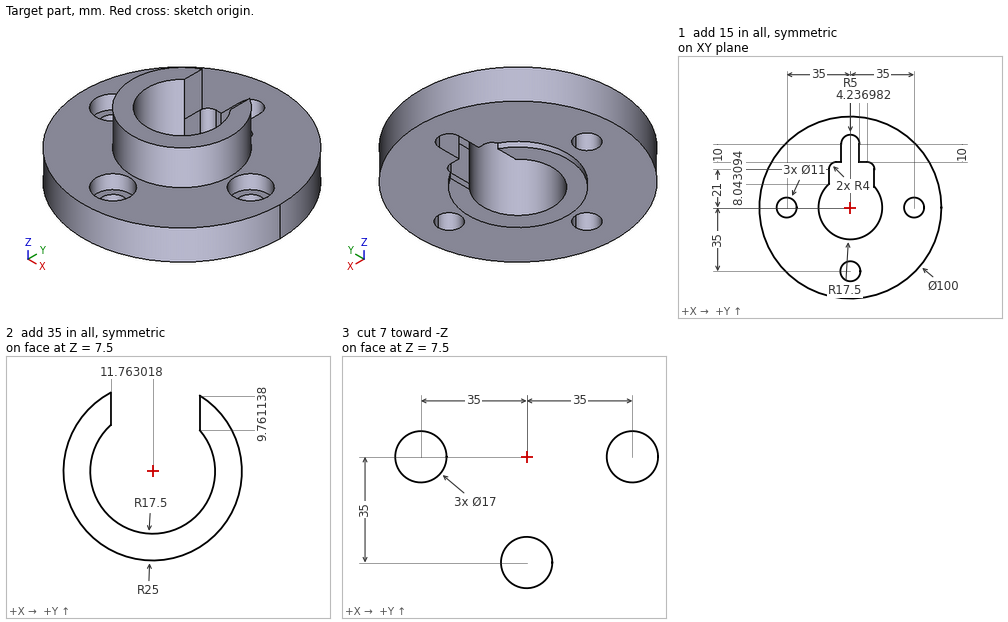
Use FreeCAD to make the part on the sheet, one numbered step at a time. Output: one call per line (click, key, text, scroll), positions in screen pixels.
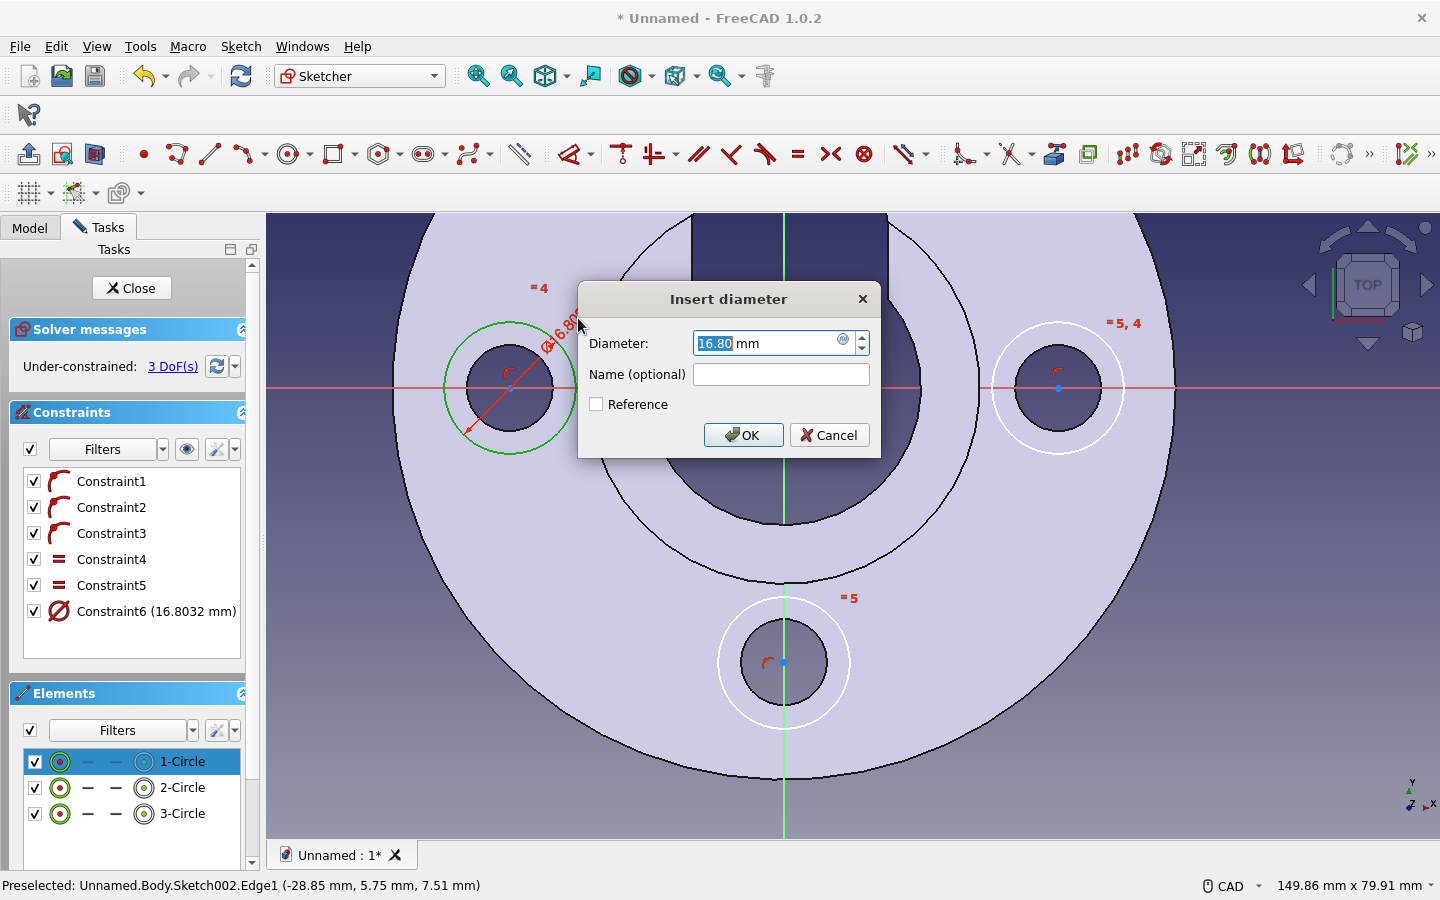
text(17)
key(Return)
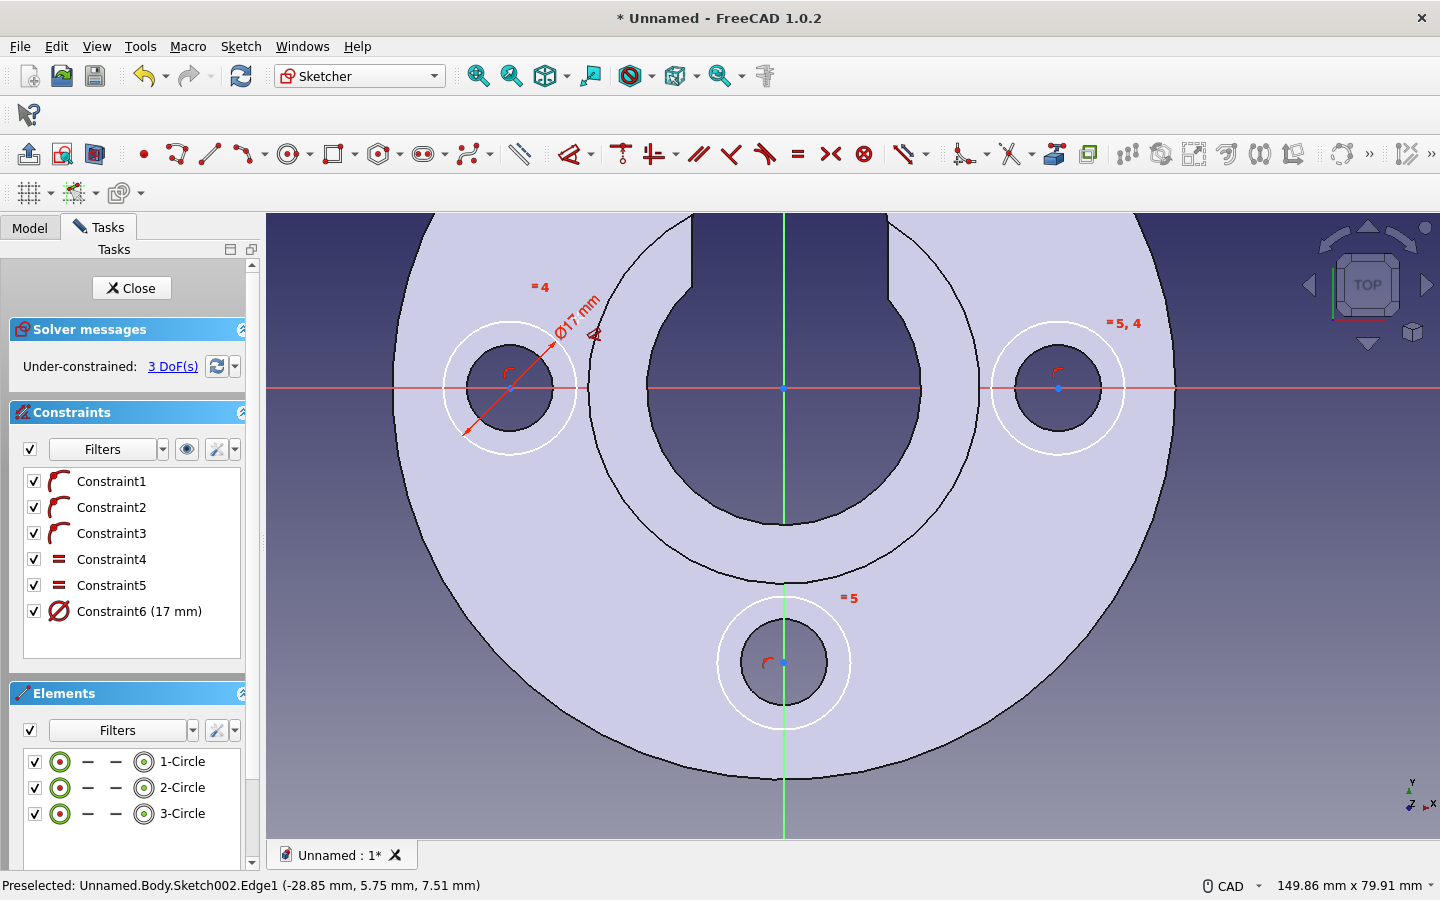
click(510, 388)
click(647, 354)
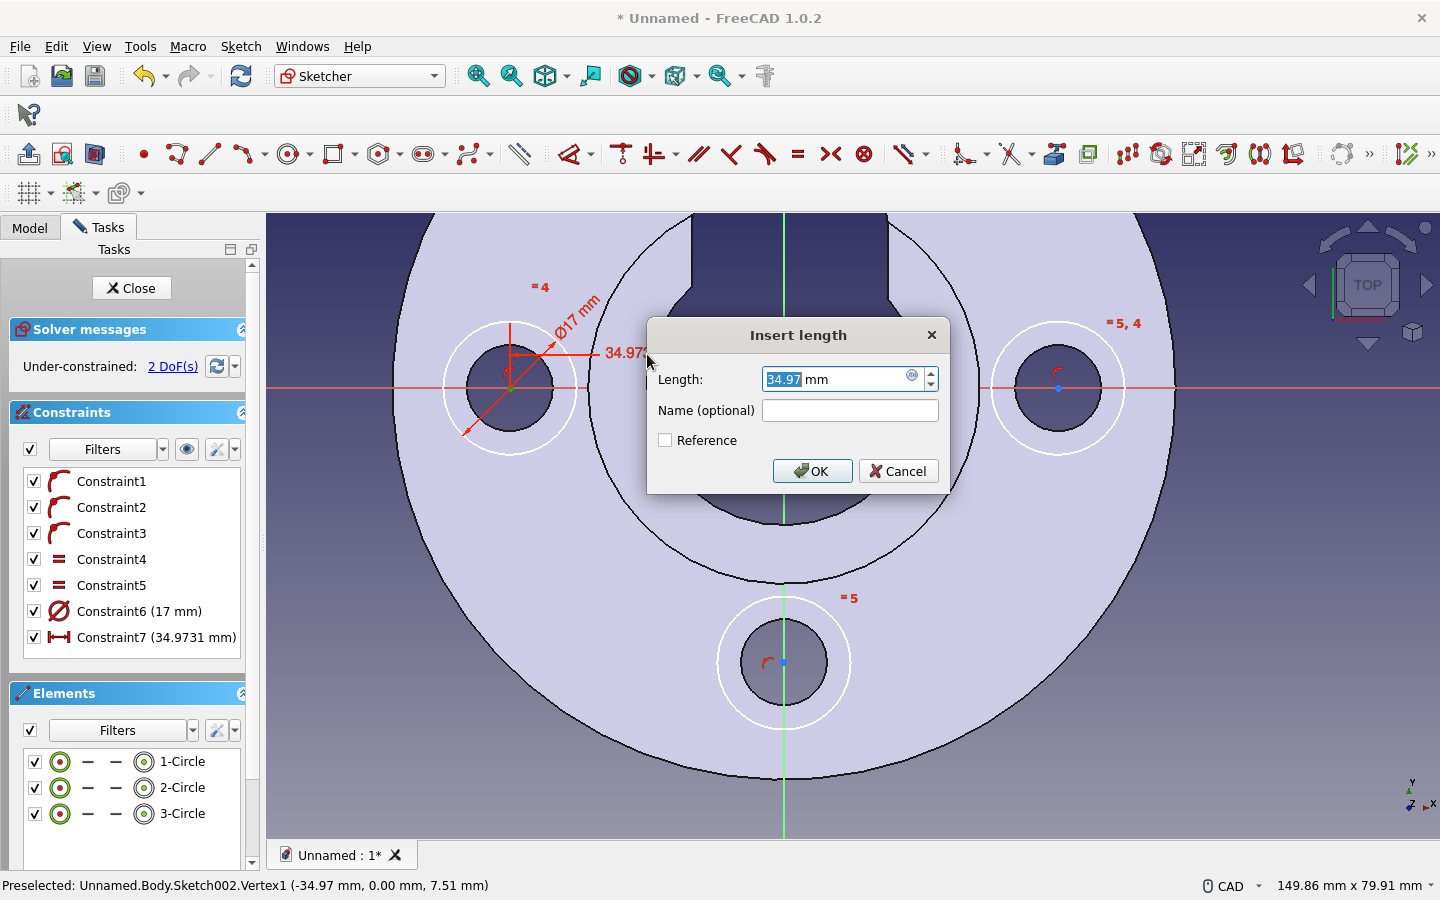
text(35)
key(Return)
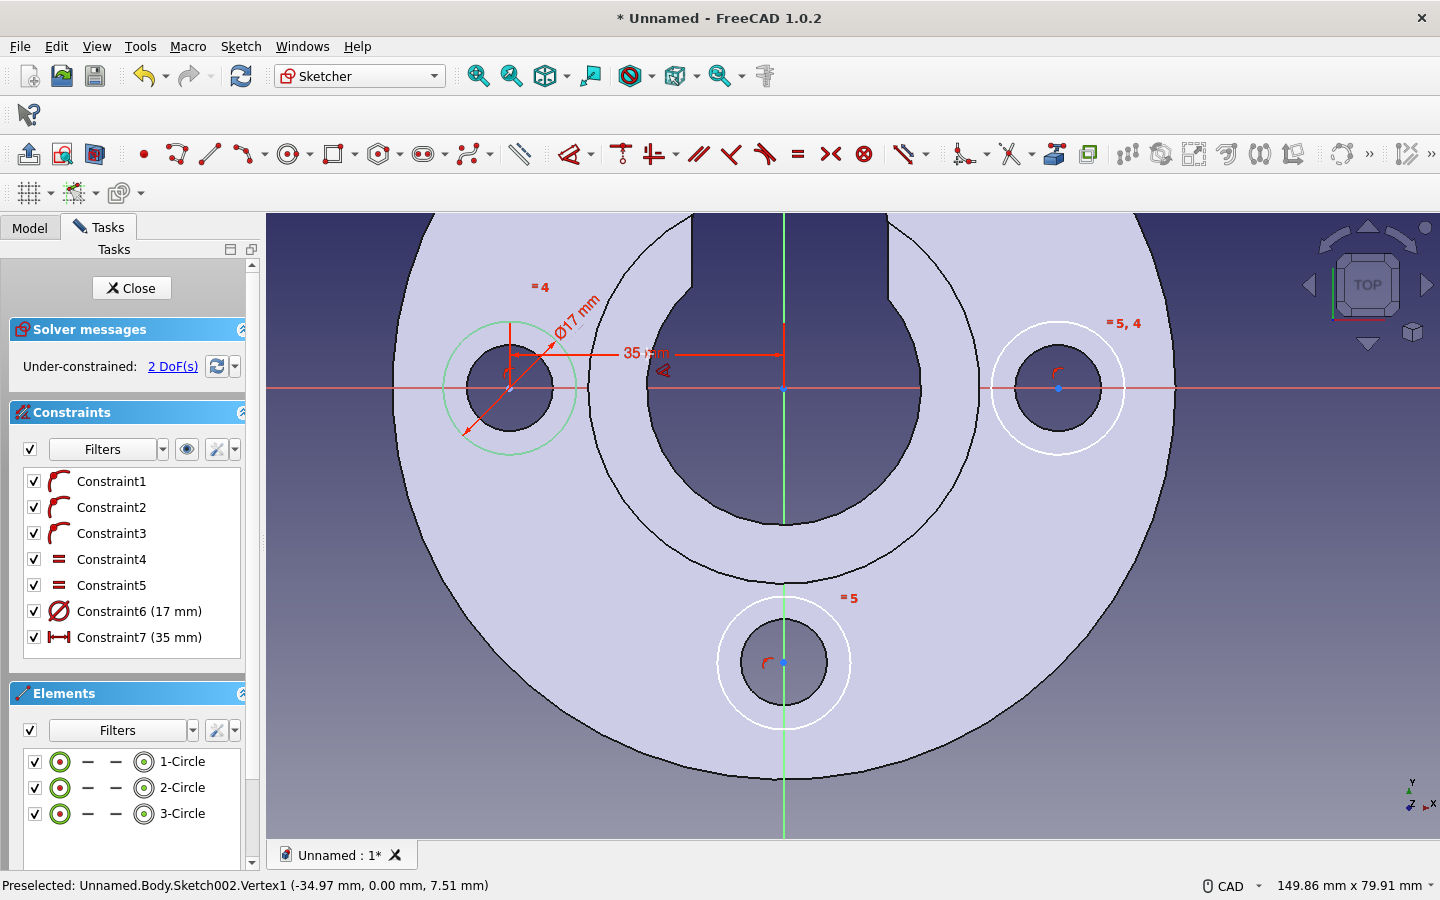
click(1058, 388)
click(921, 354)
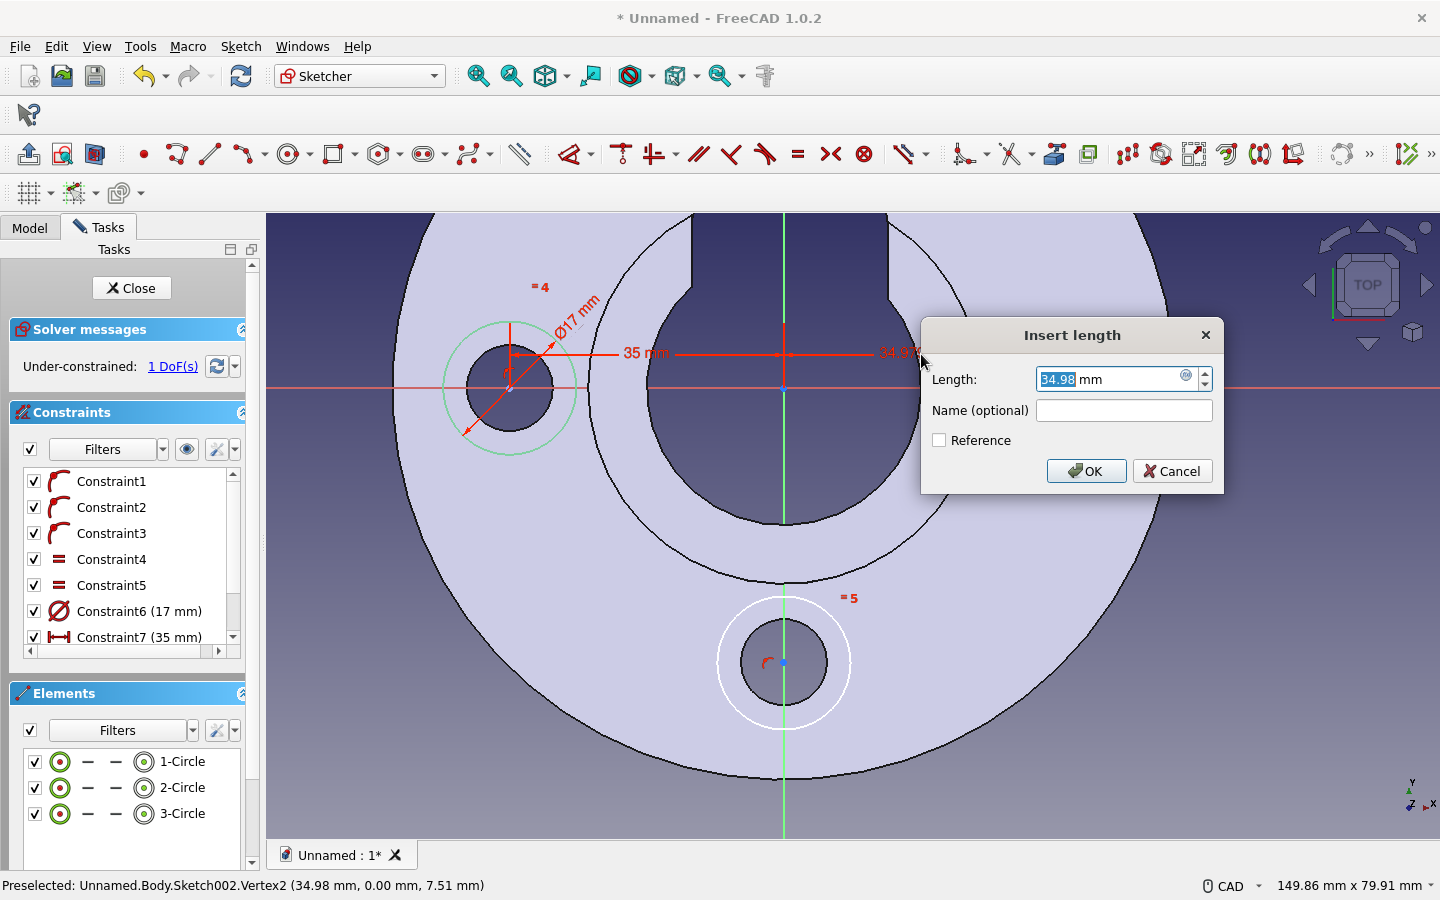
text(35)
key(Return)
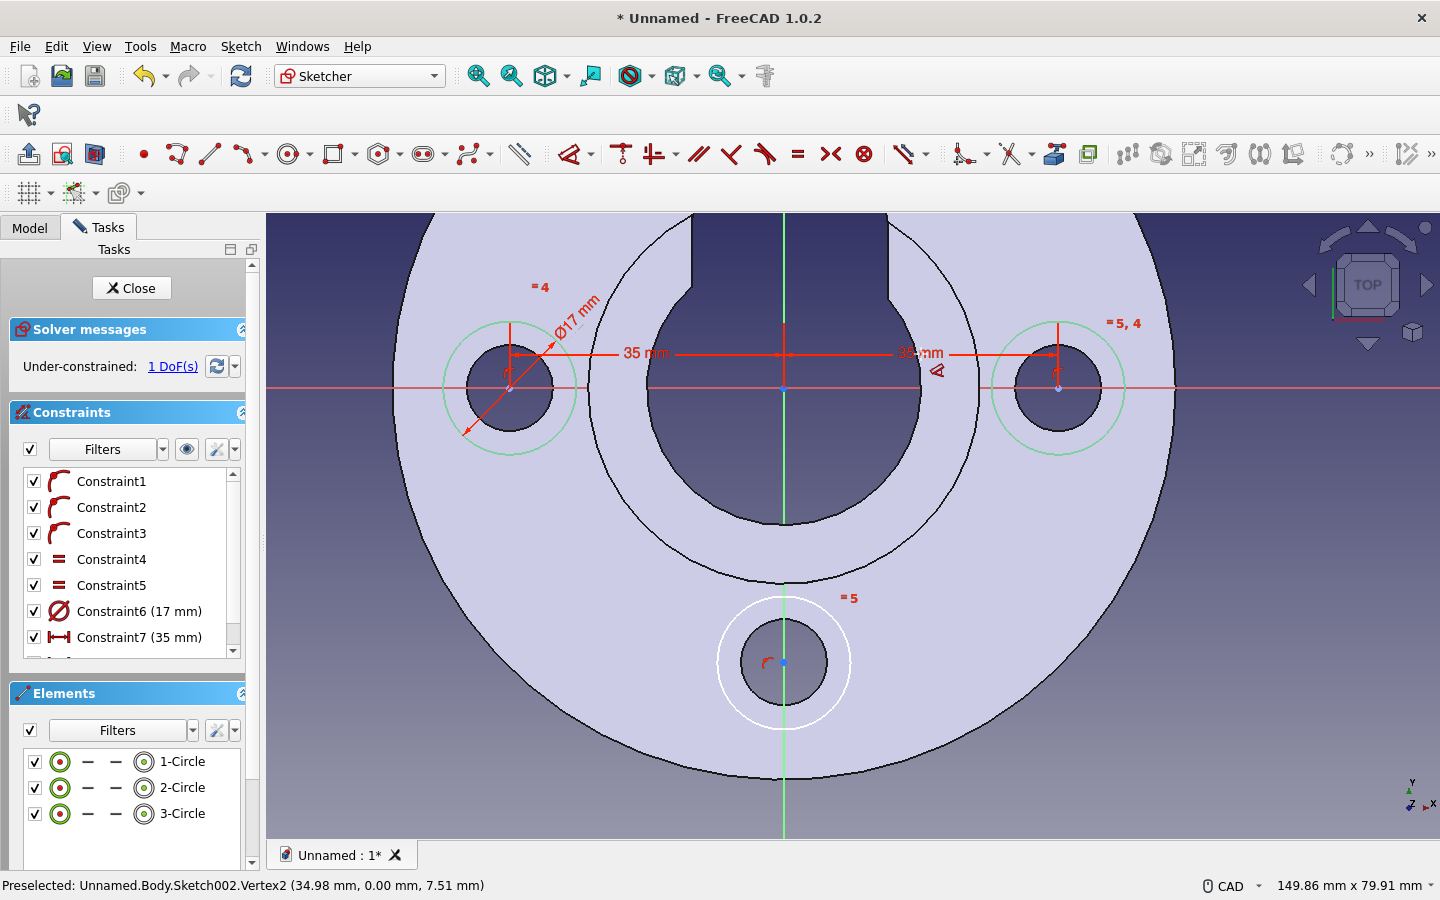
click(784, 663)
click(818, 526)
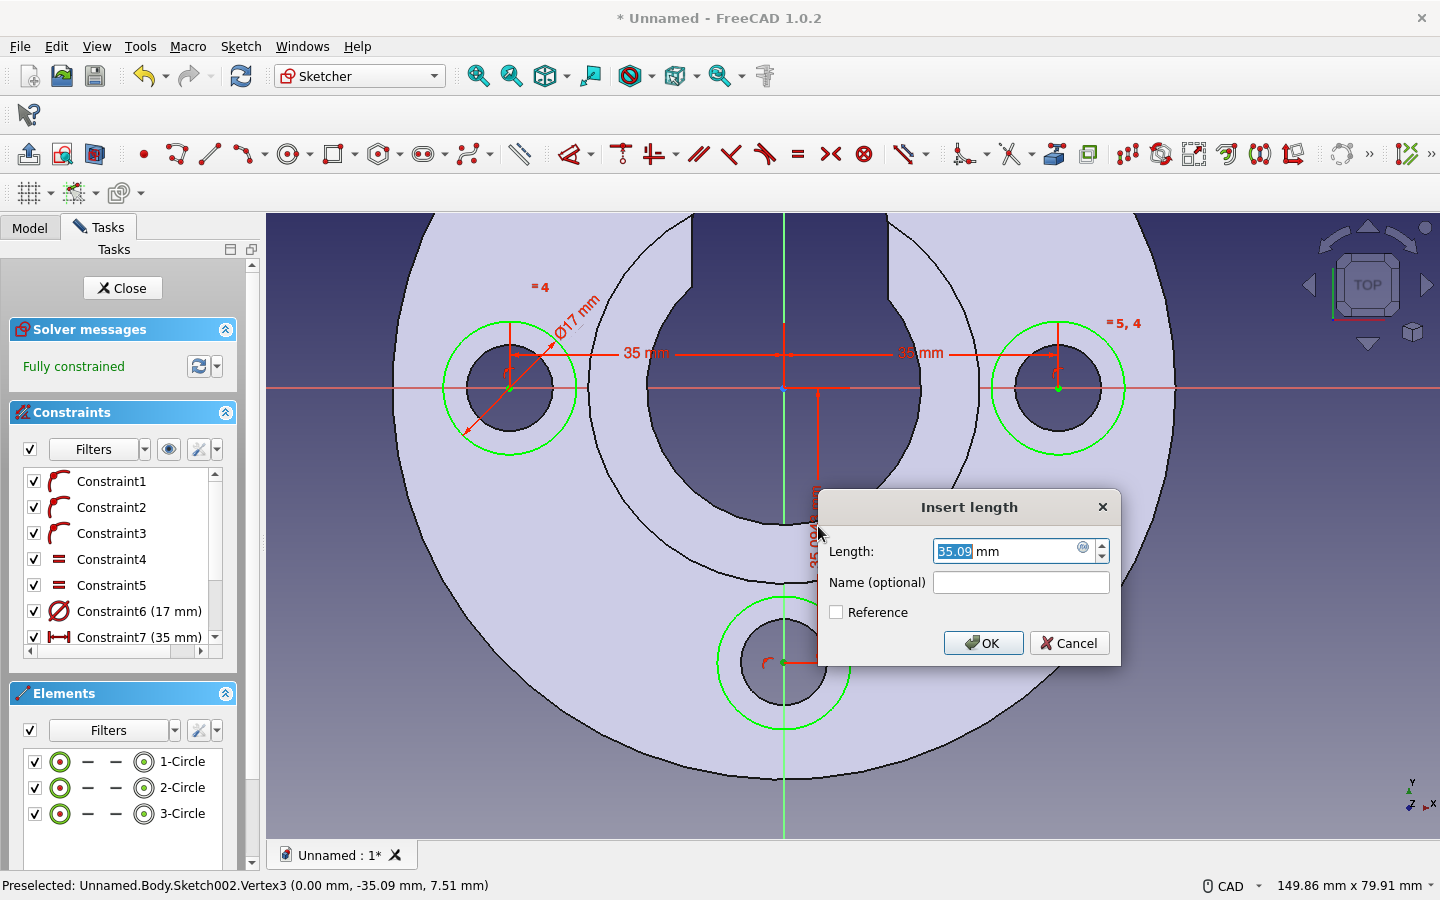
text(35)
key(Return)
key(Escape)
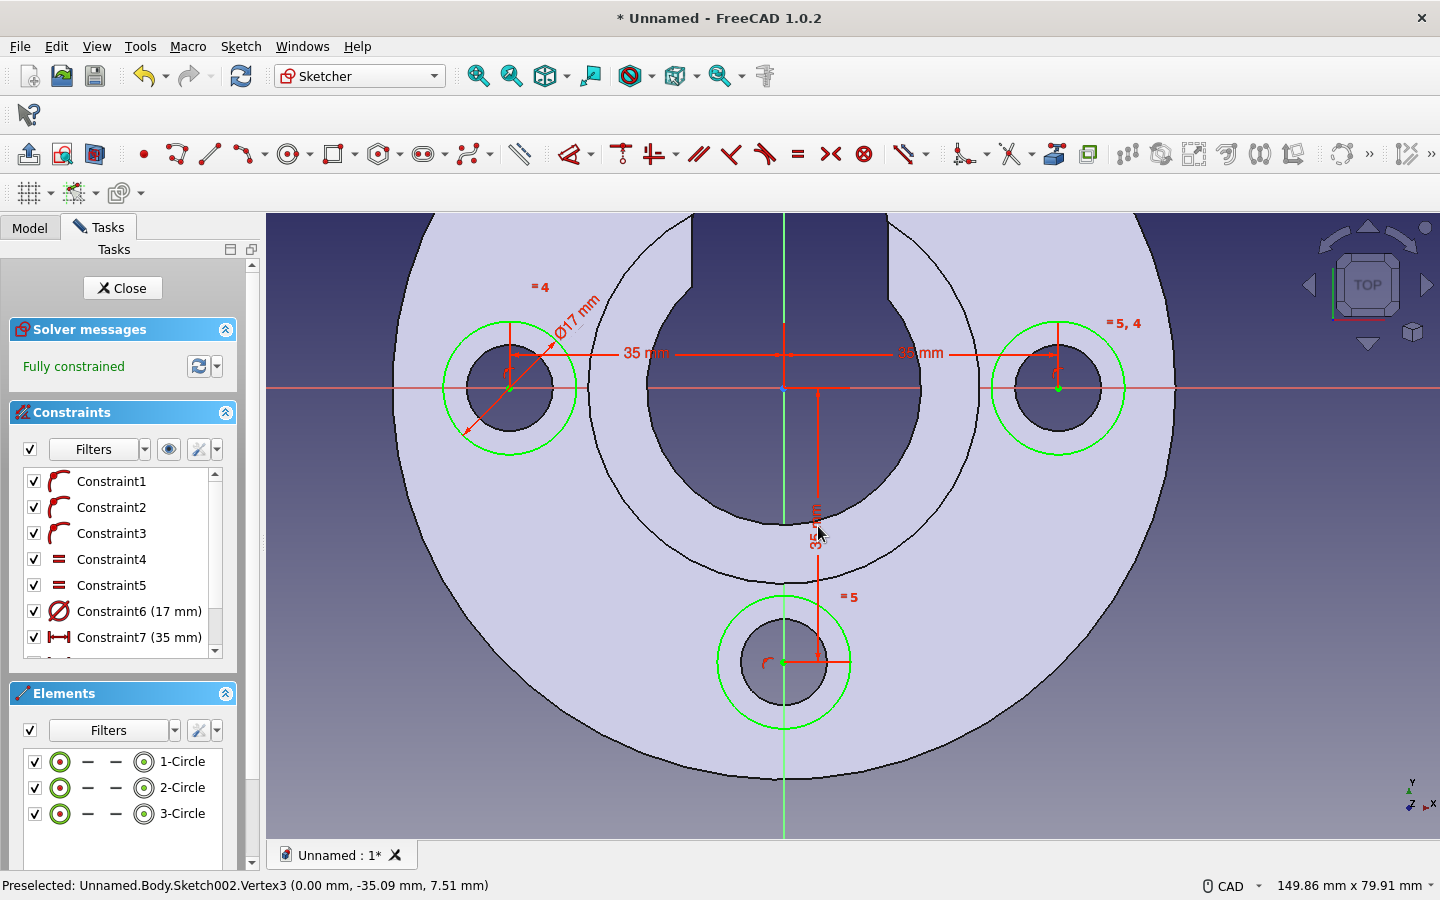
click(123, 288)